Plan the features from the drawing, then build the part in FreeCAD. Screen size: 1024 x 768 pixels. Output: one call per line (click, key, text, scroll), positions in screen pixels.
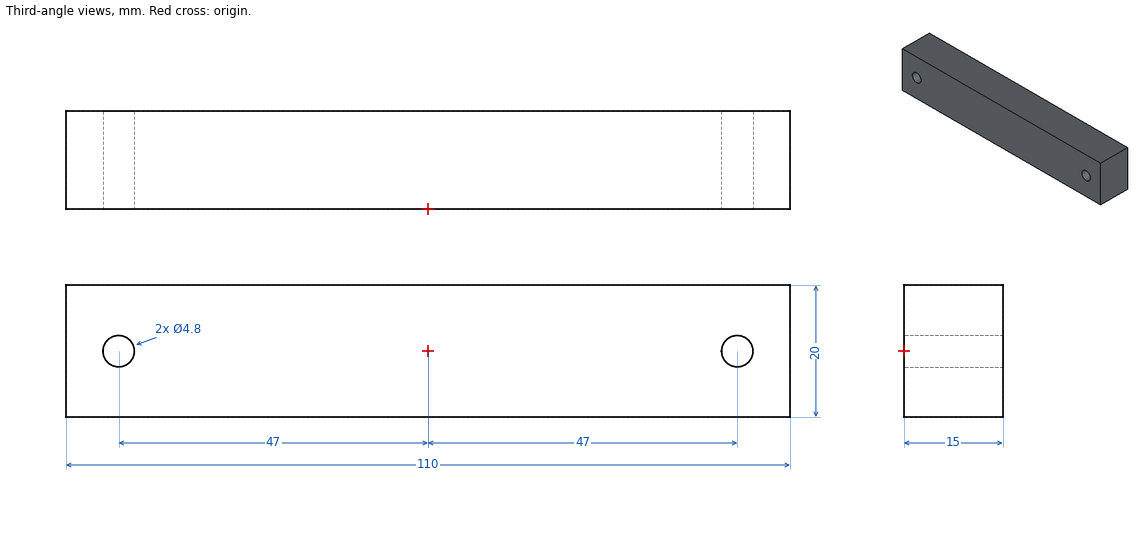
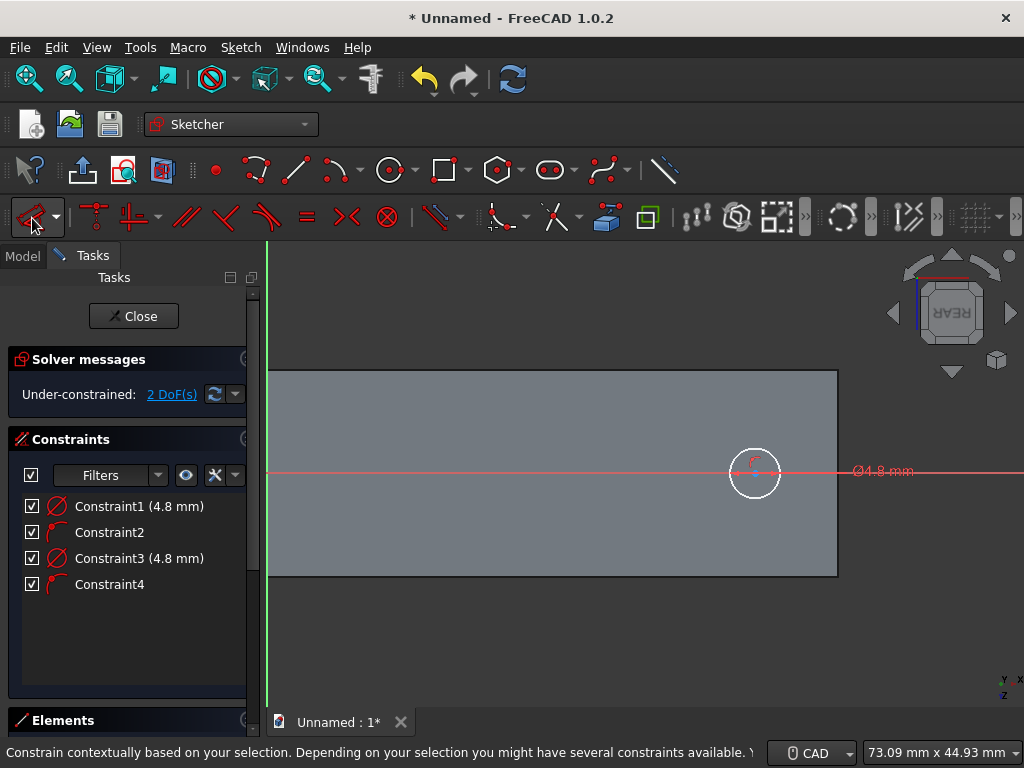
scroll(757, 474, down, 5)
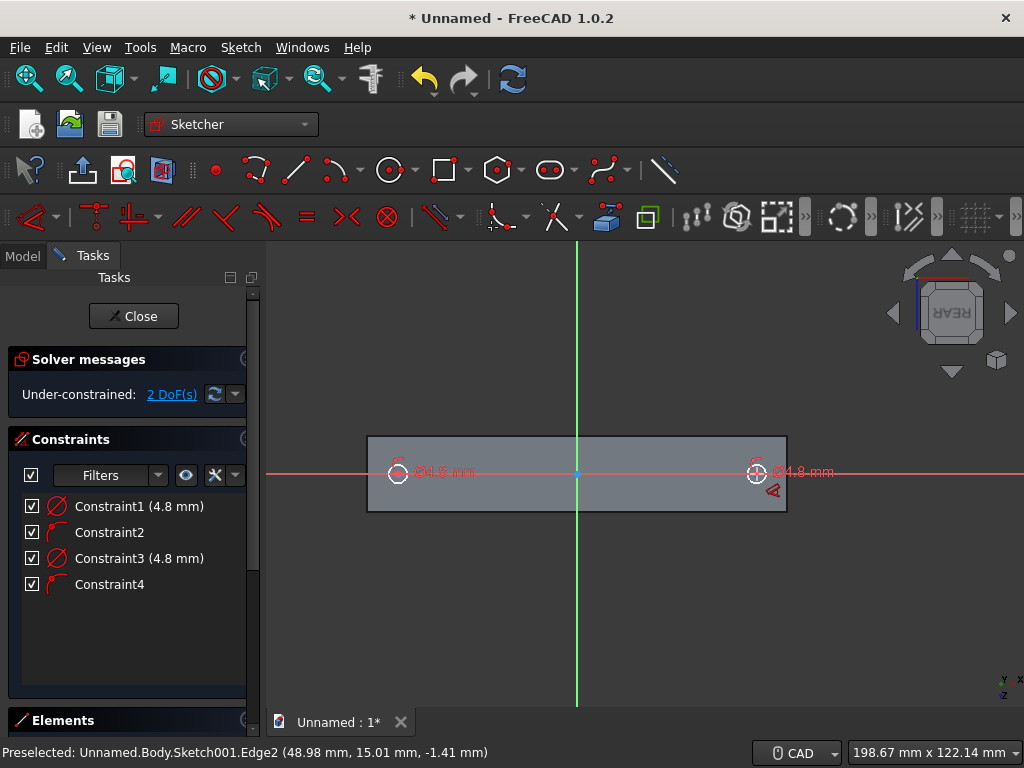
click(398, 474)
click(488, 508)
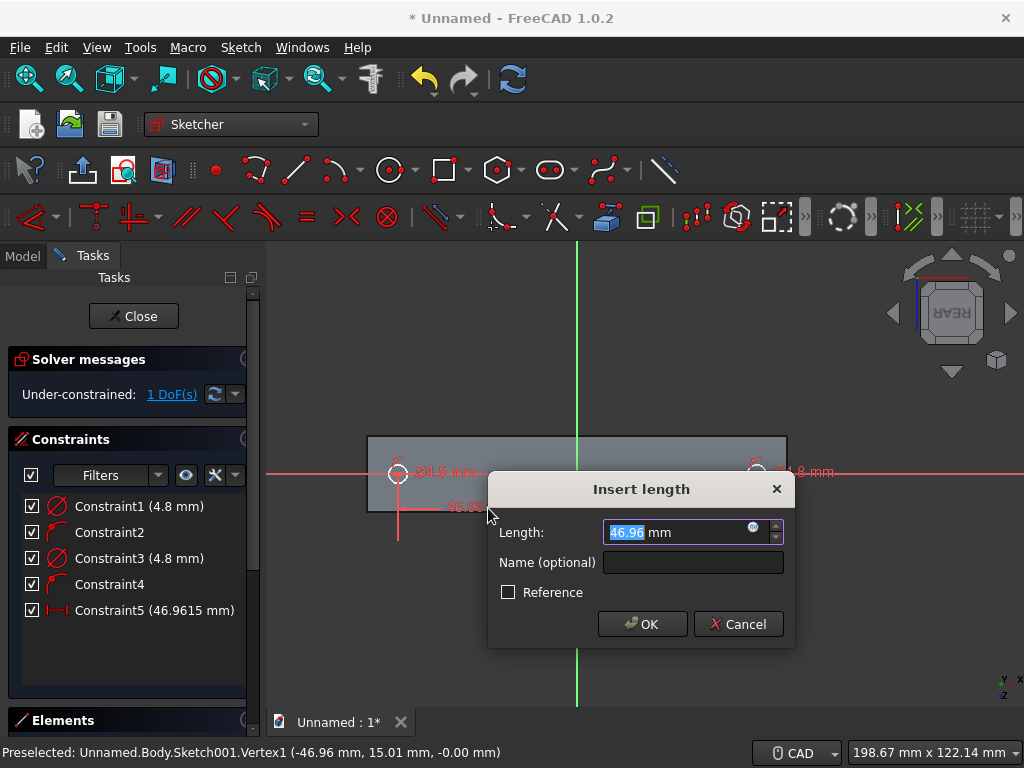
text(47)
key(Return)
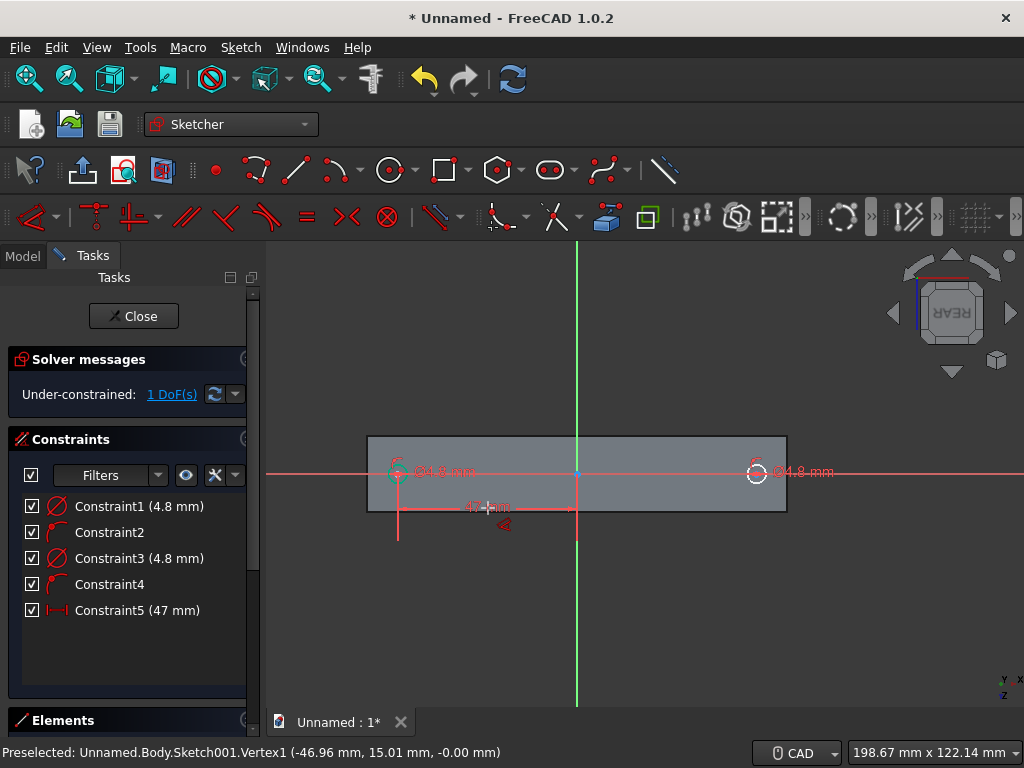
click(757, 474)
click(667, 508)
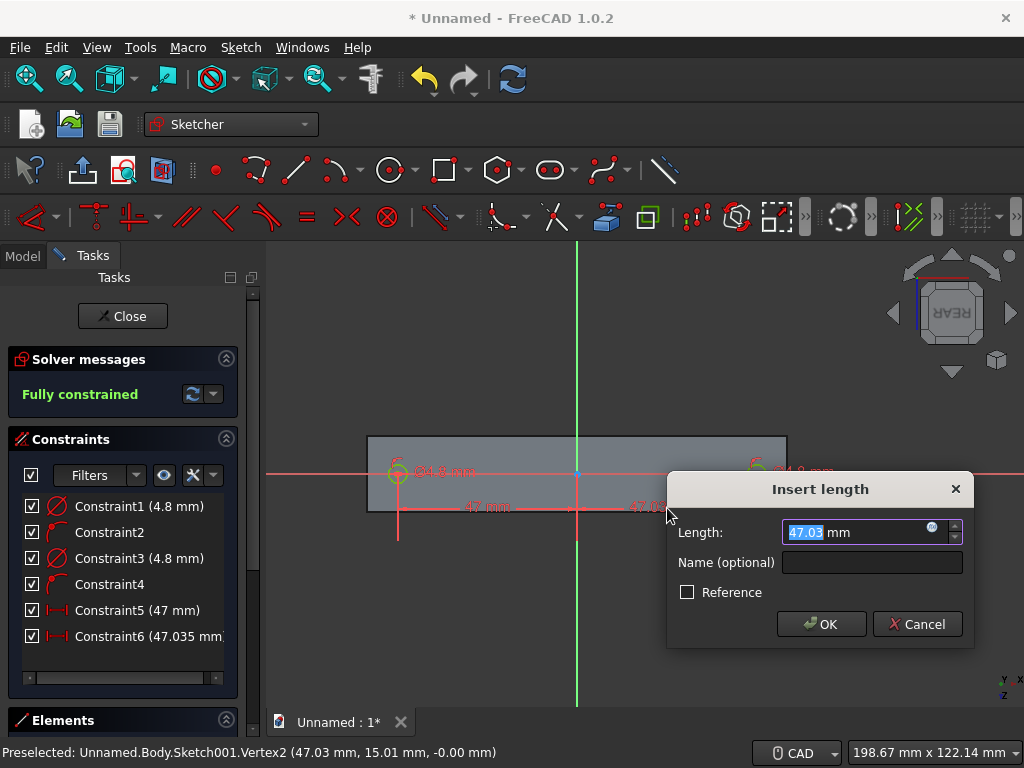
text(47)
key(Return)
key(Escape)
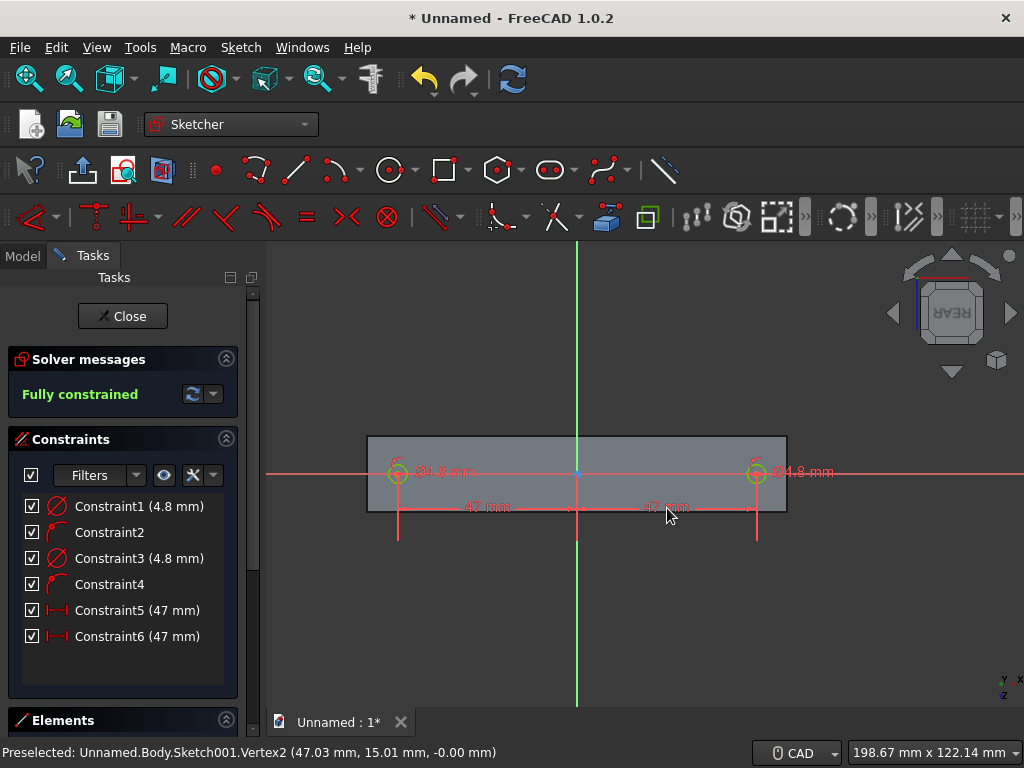
click(123, 316)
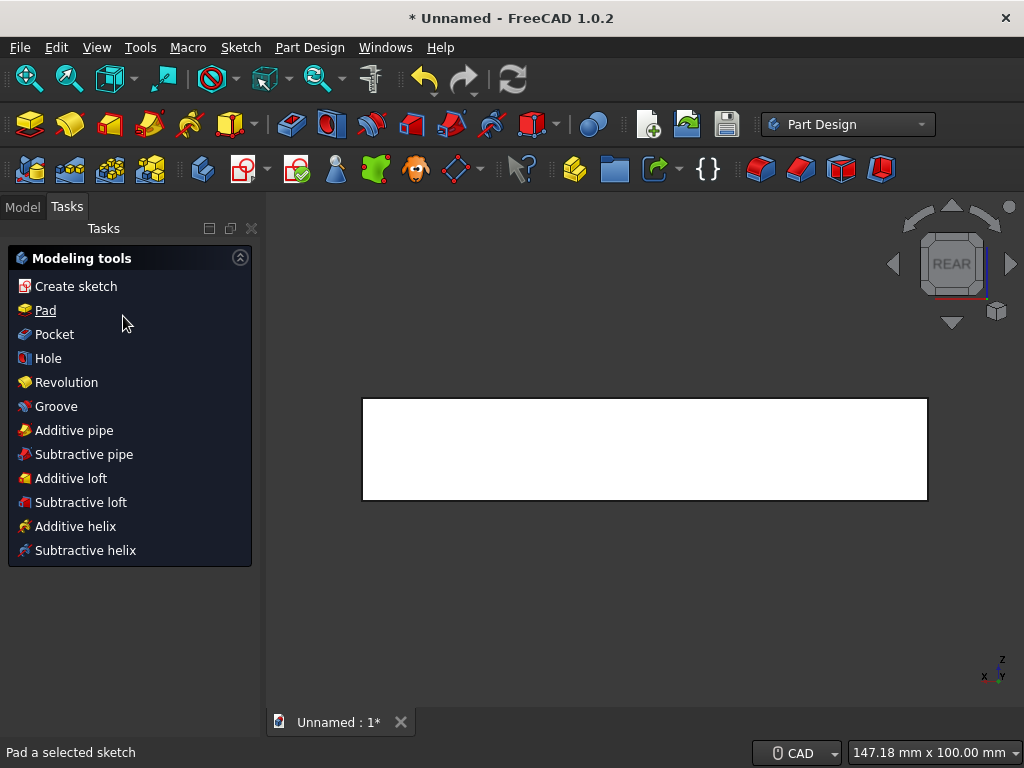
click(292, 124)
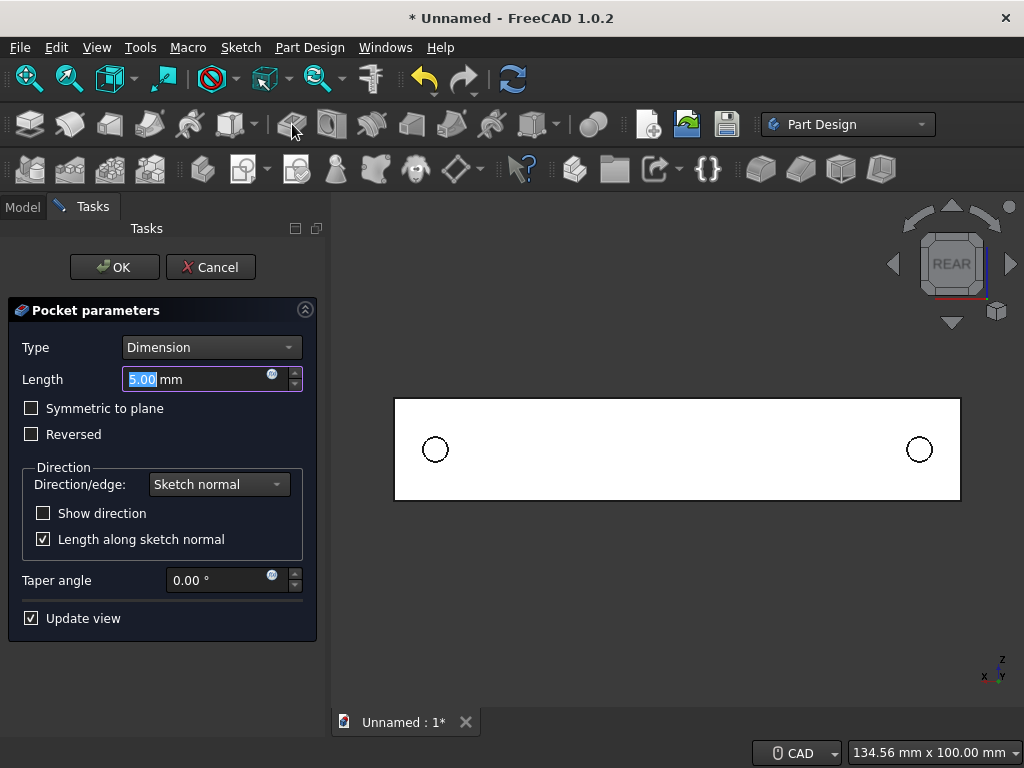
click(212, 348)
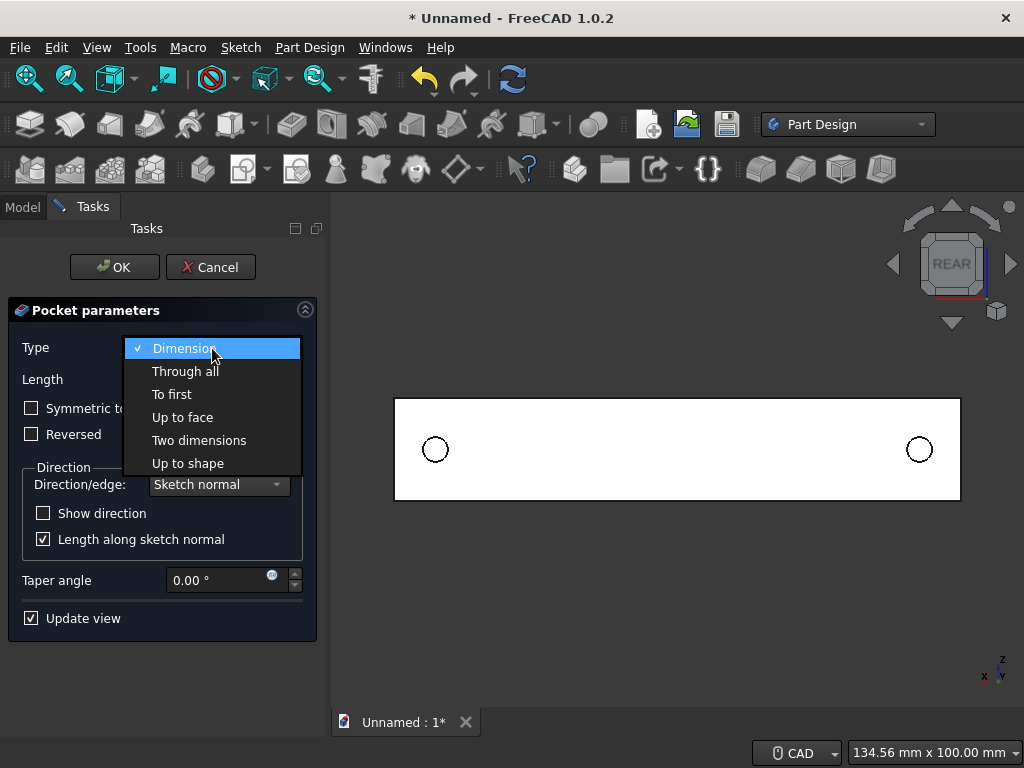
click(212, 372)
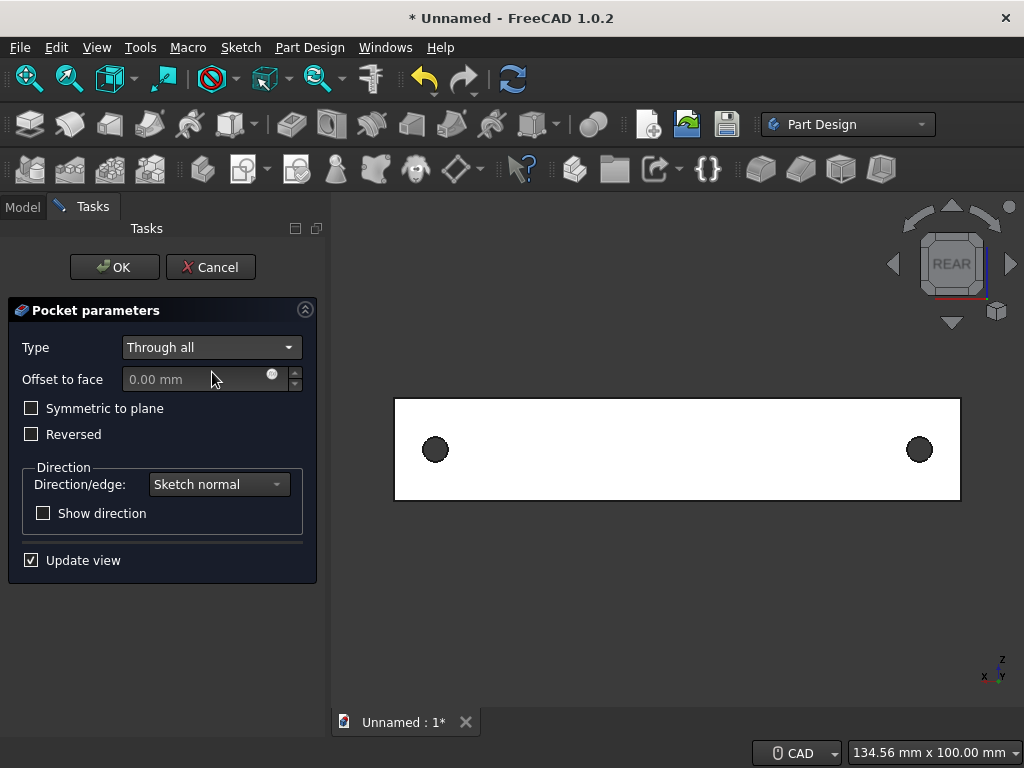
click(115, 267)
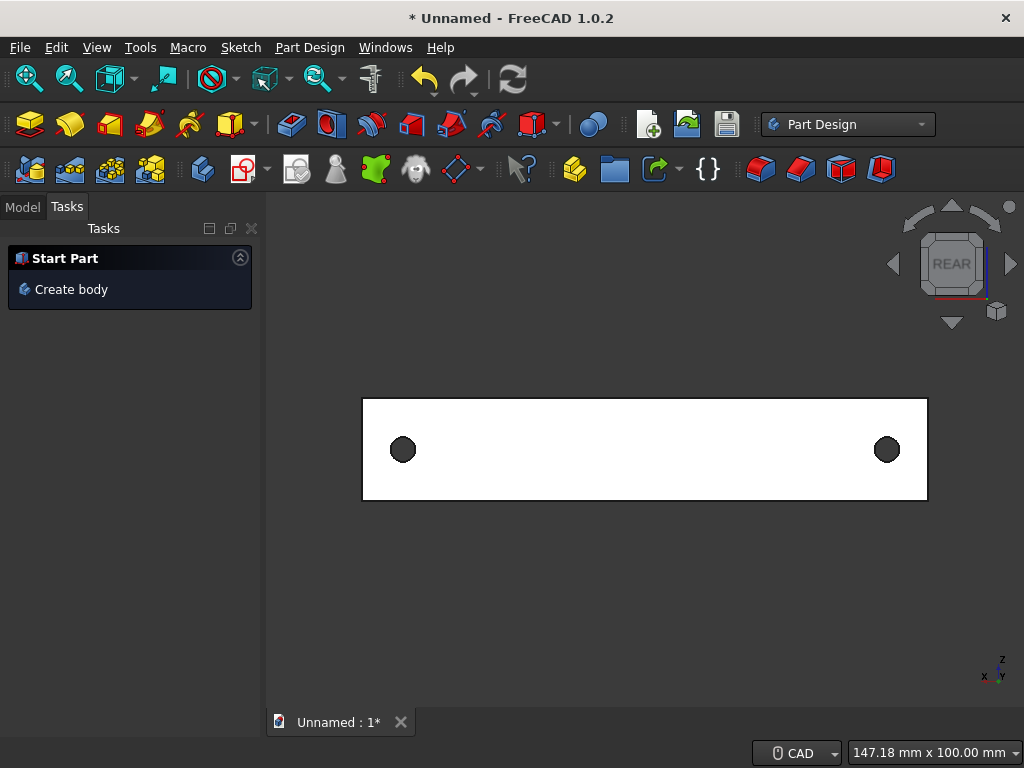
key(0)